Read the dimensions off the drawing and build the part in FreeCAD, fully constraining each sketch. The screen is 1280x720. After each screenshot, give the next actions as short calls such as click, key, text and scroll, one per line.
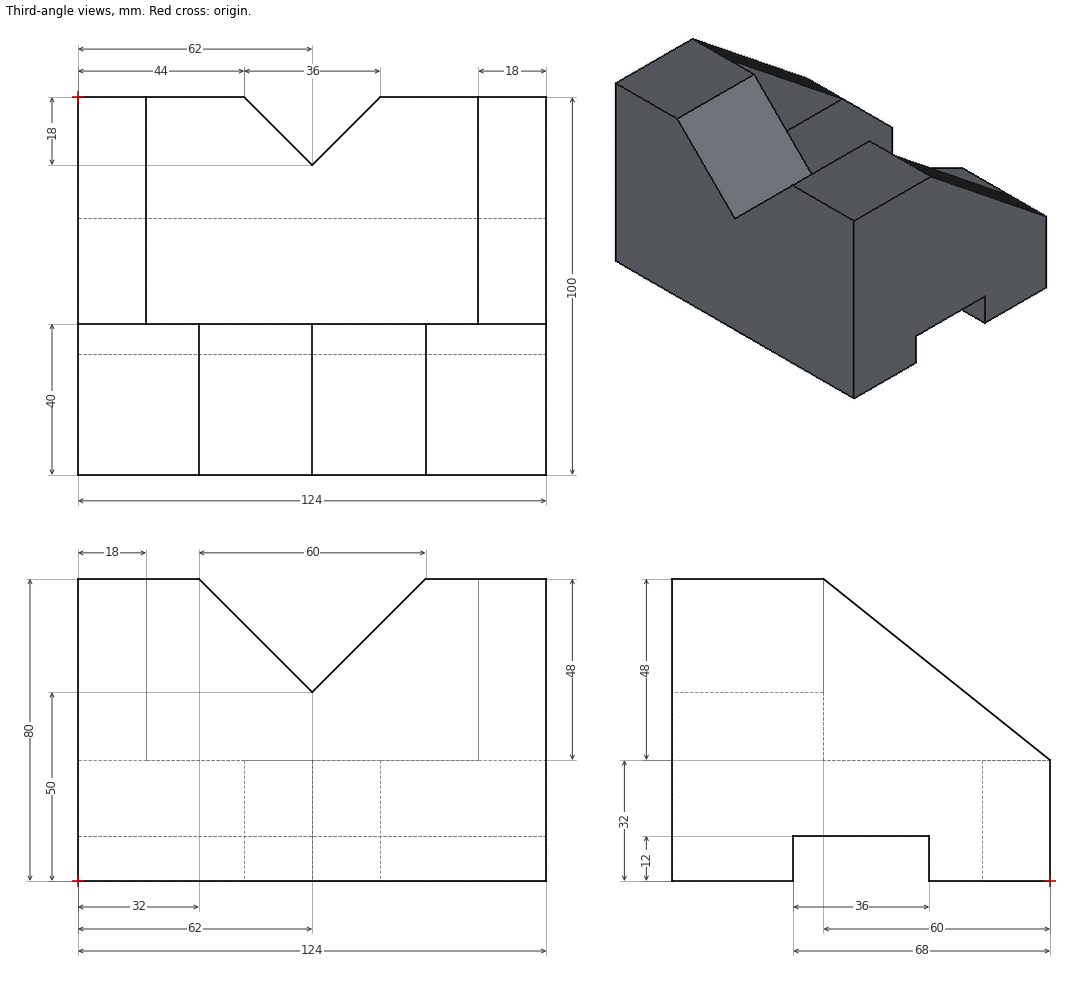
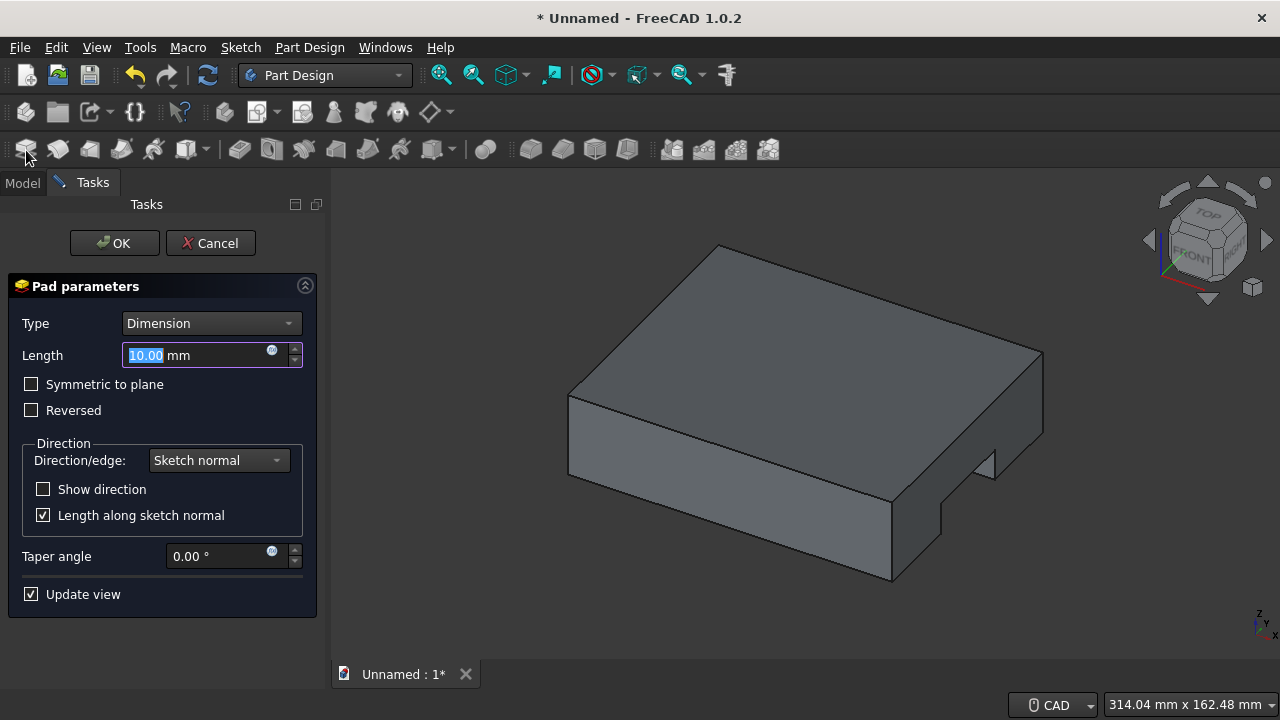
text(40)
key(Tab)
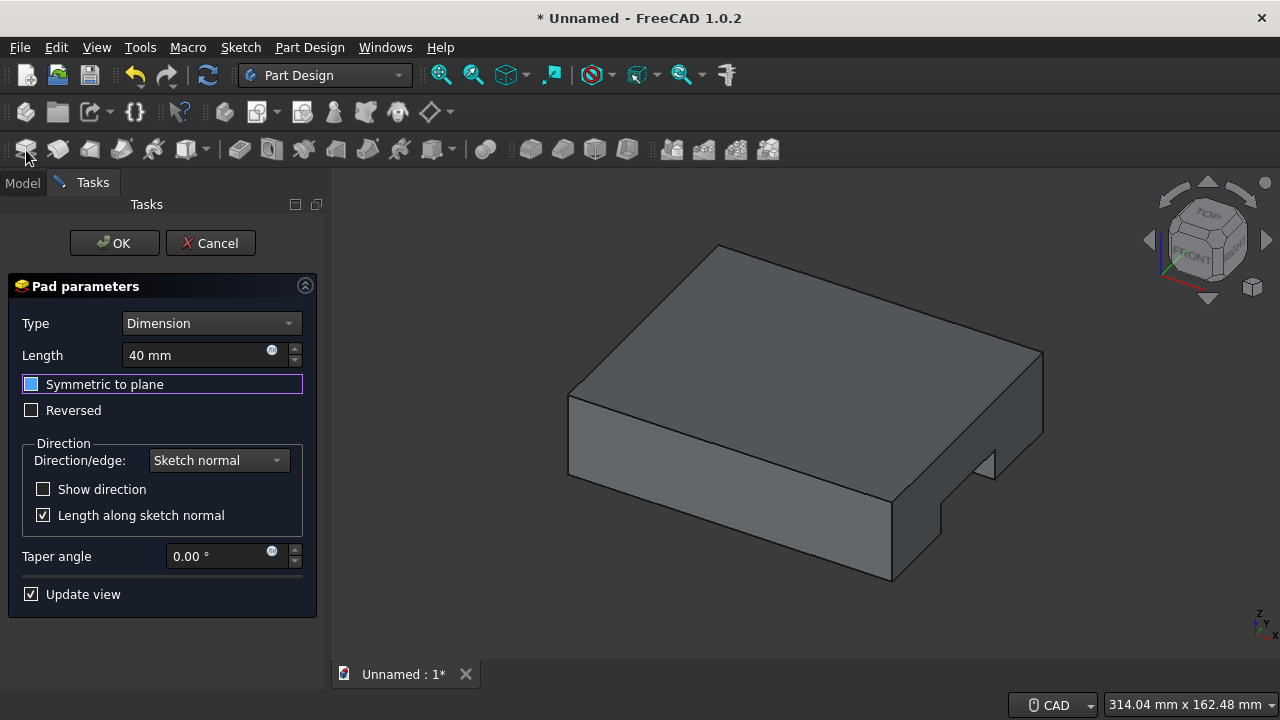
click(30, 410)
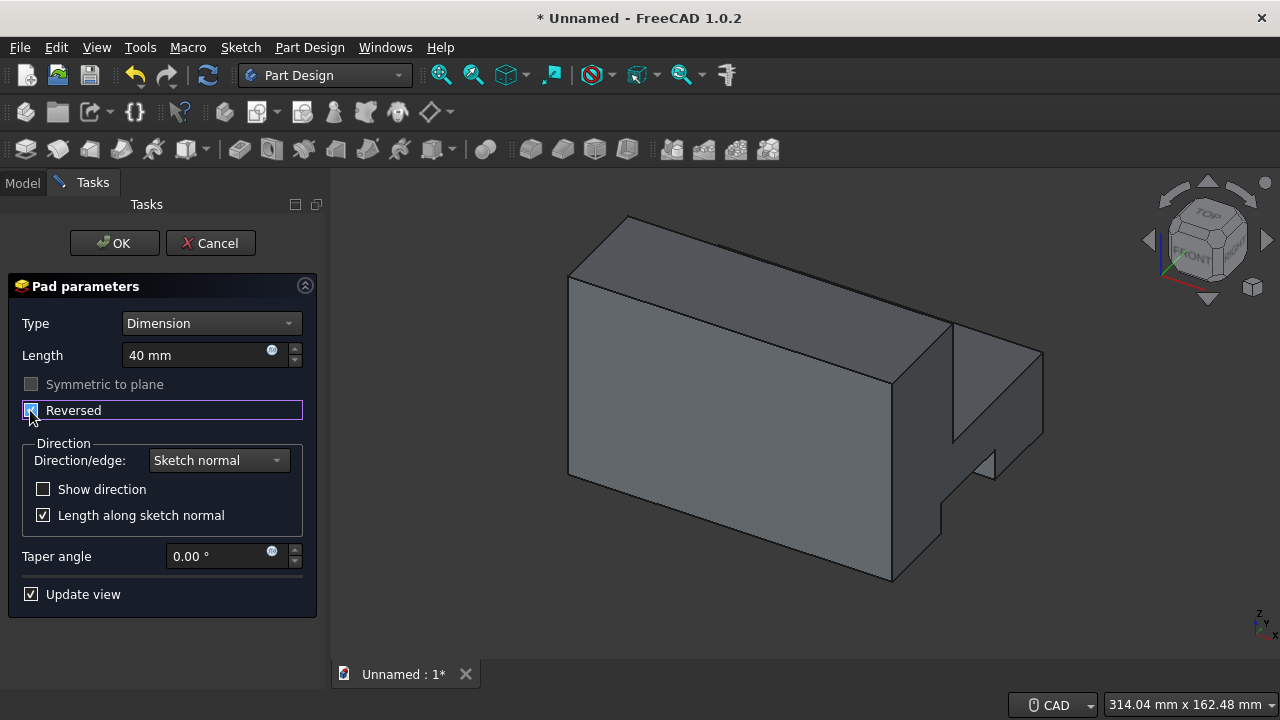
click(115, 243)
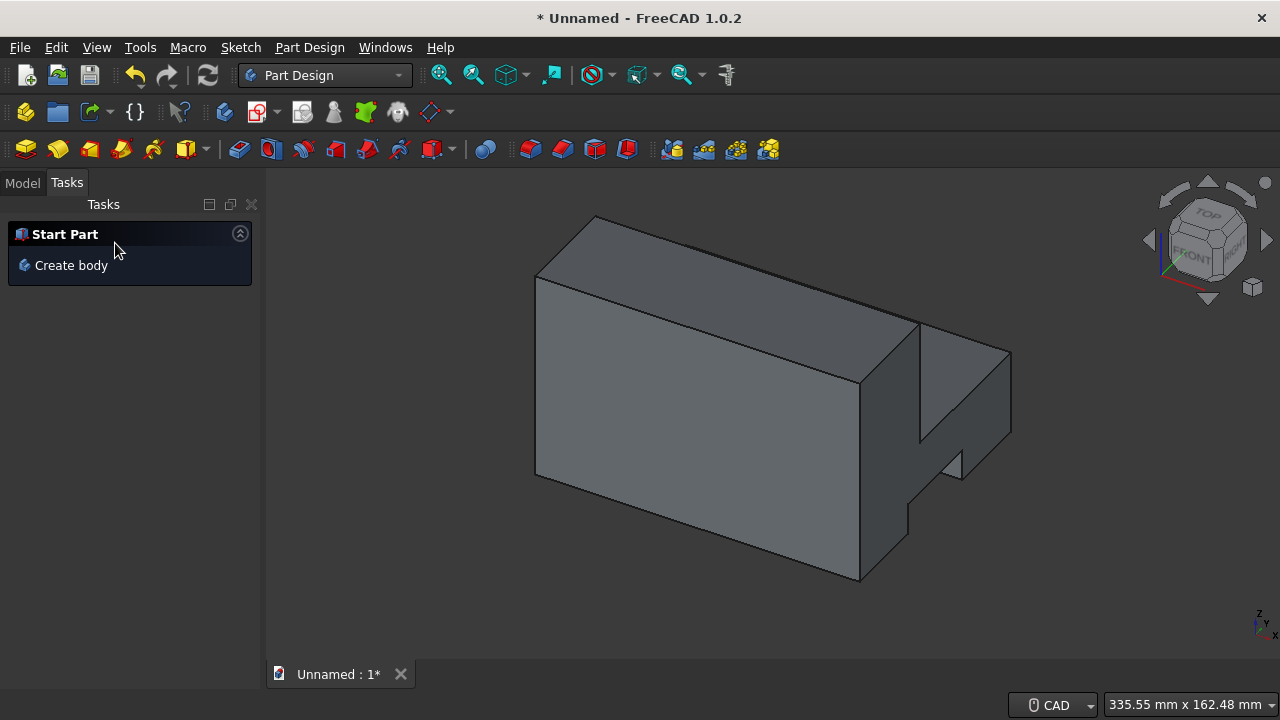
click(442, 76)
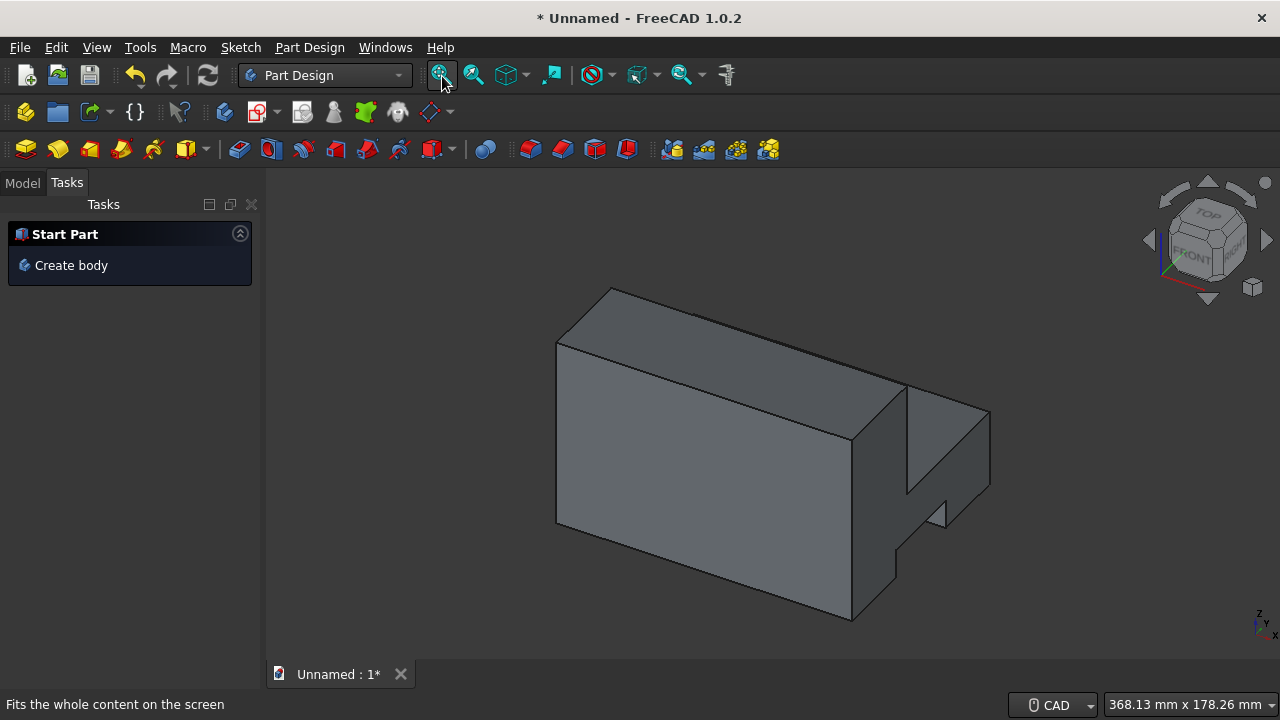
click(882, 526)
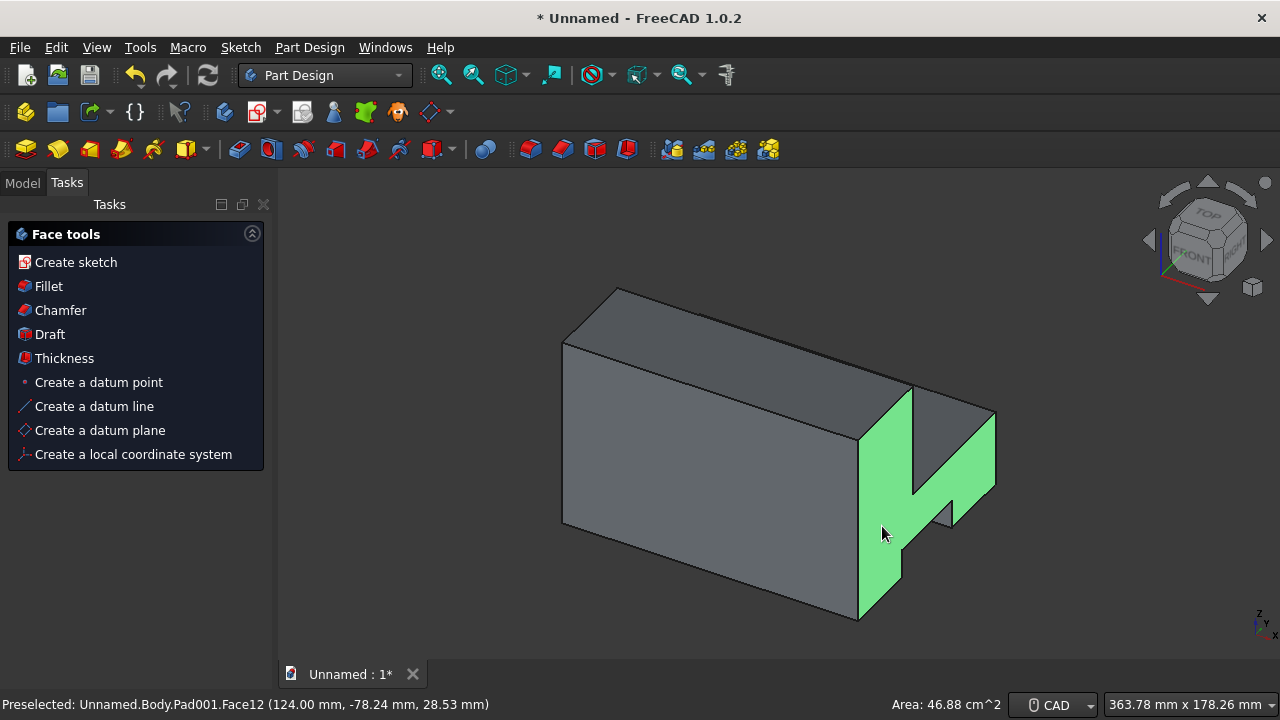
click(258, 112)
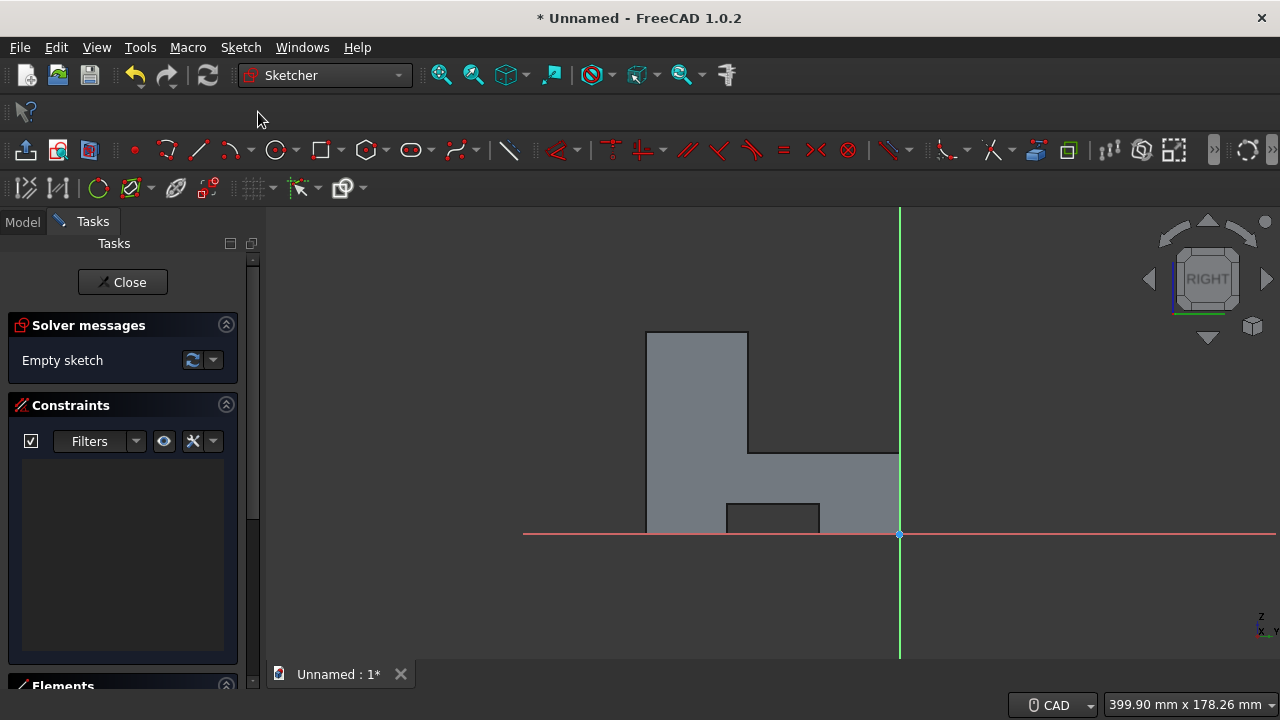
scroll(1066, 433, up, 2)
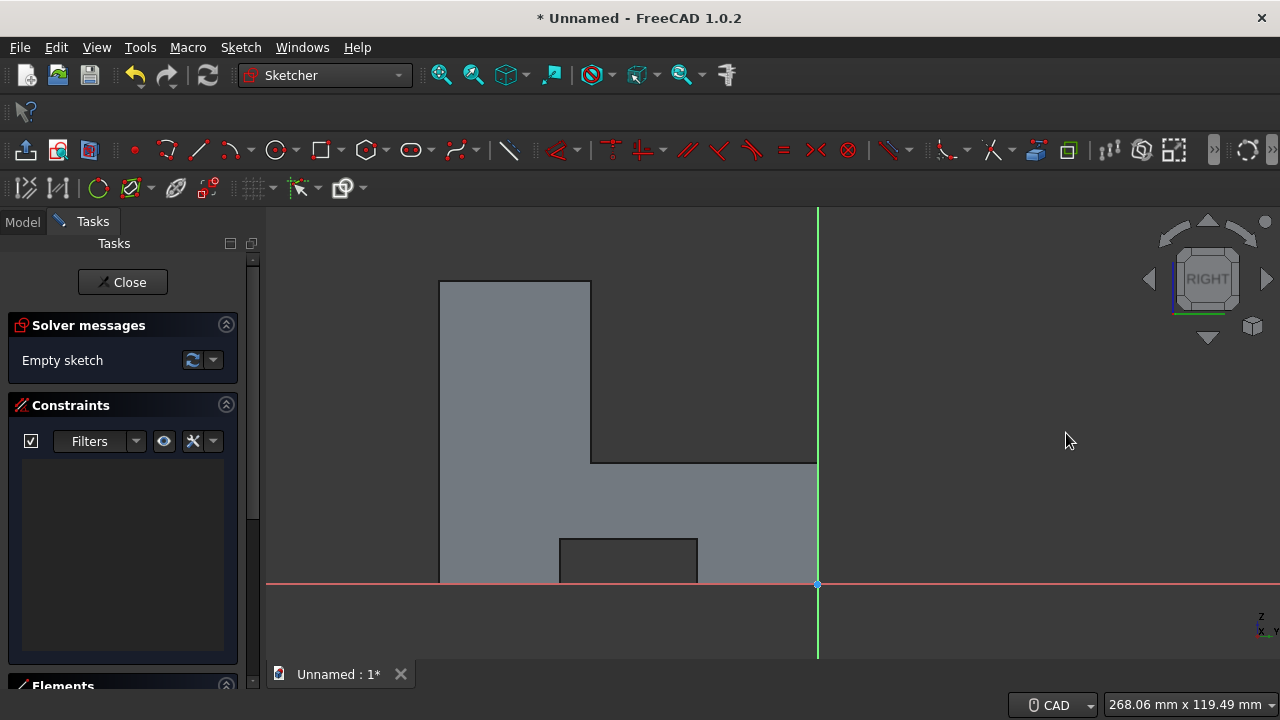
click(168, 150)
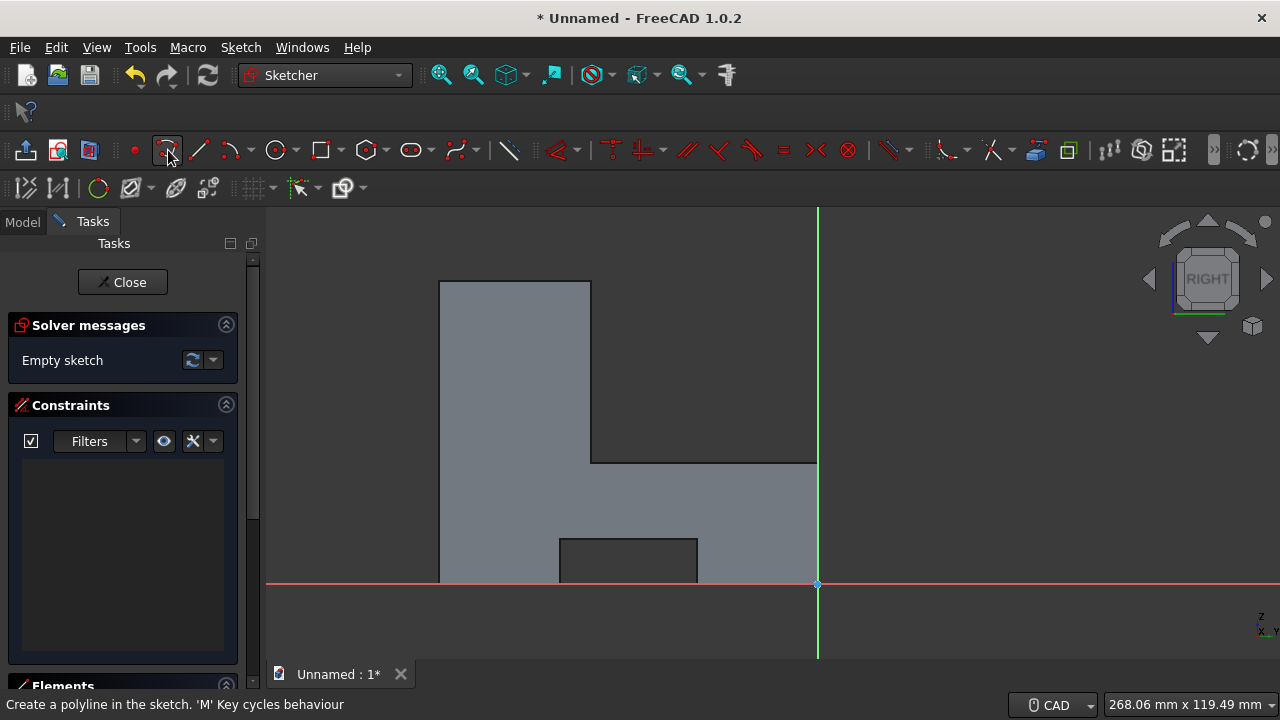
click(818, 463)
click(591, 281)
click(591, 463)
click(818, 464)
key(Escape)
key(Escape)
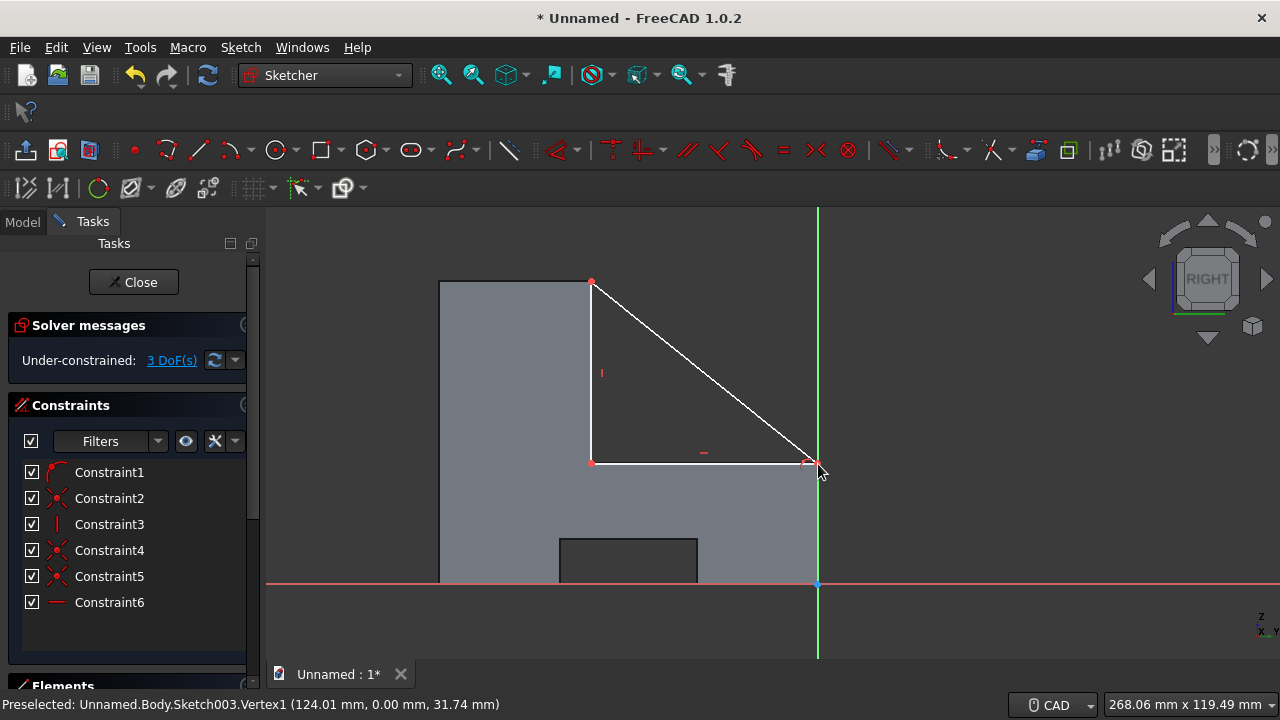
click(556, 150)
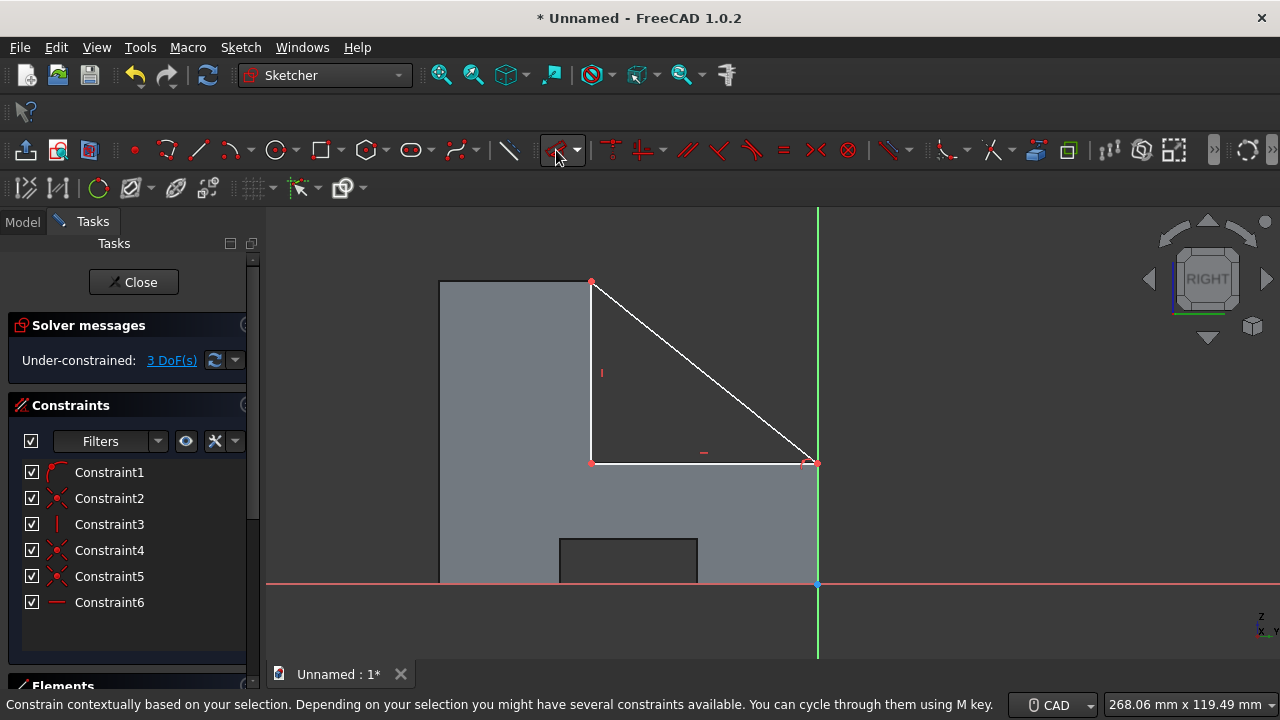
click(591, 337)
click(557, 373)